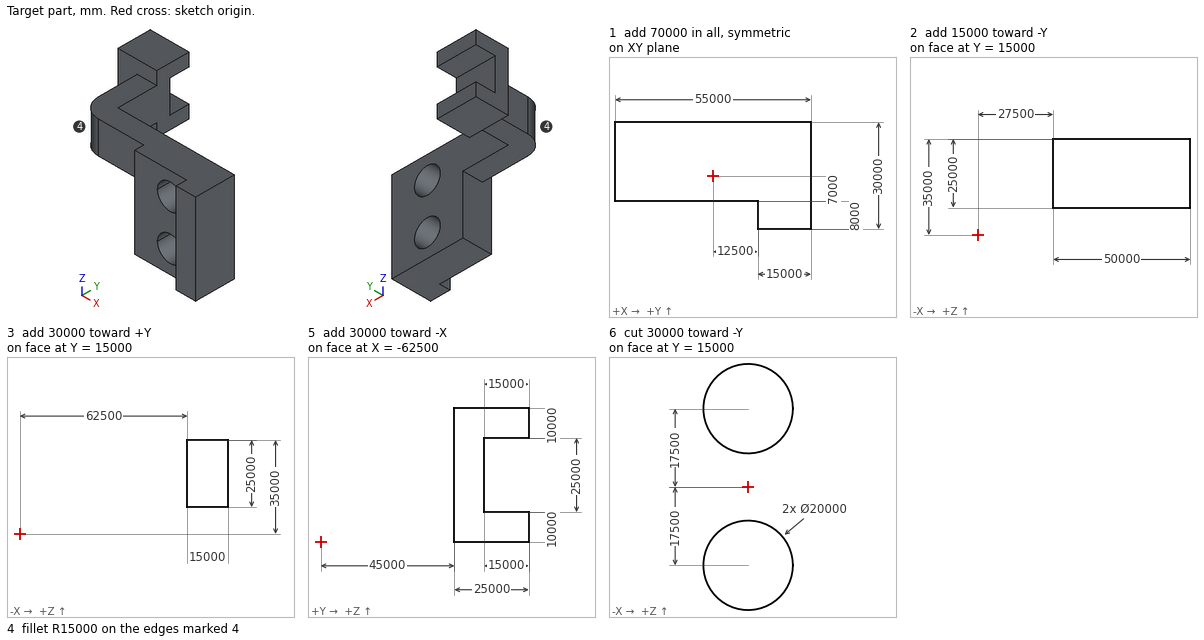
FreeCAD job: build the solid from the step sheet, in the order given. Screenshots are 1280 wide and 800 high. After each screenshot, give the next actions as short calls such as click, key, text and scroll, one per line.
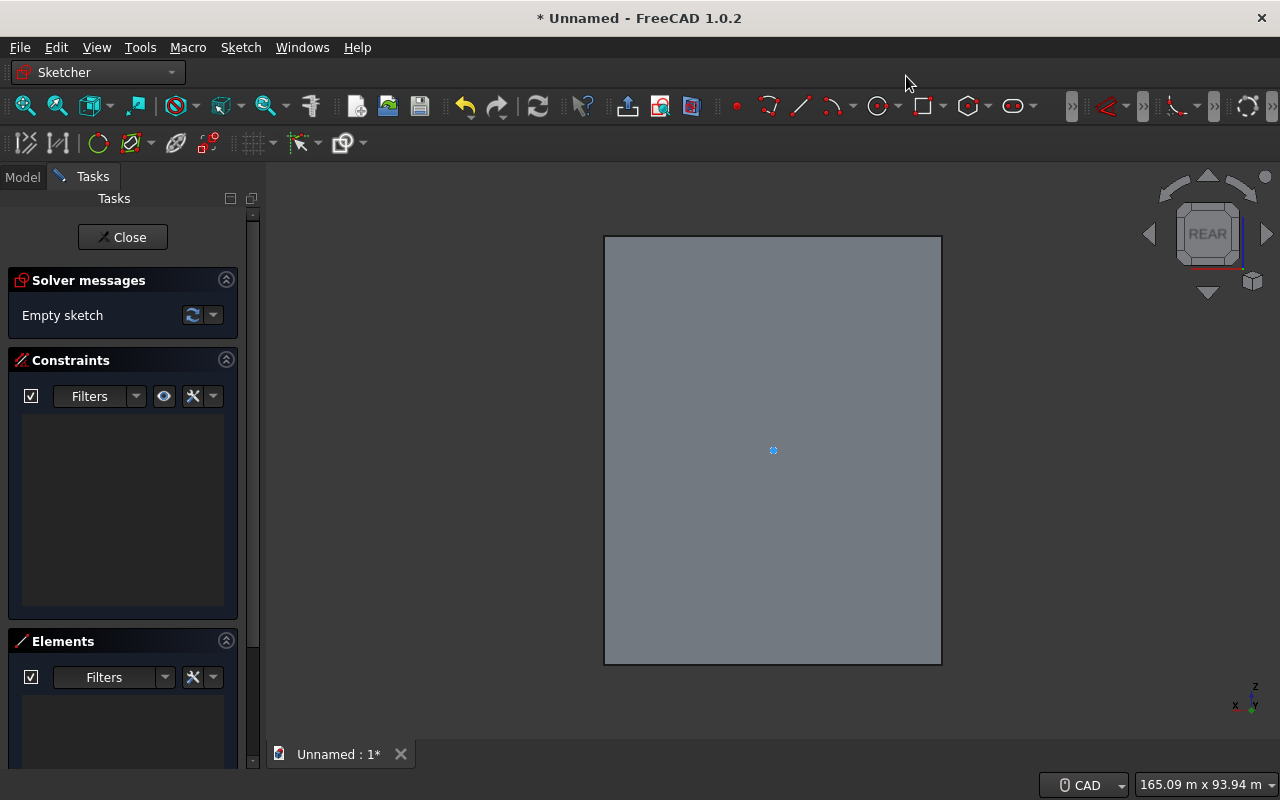
scroll(294, 711, down, 1)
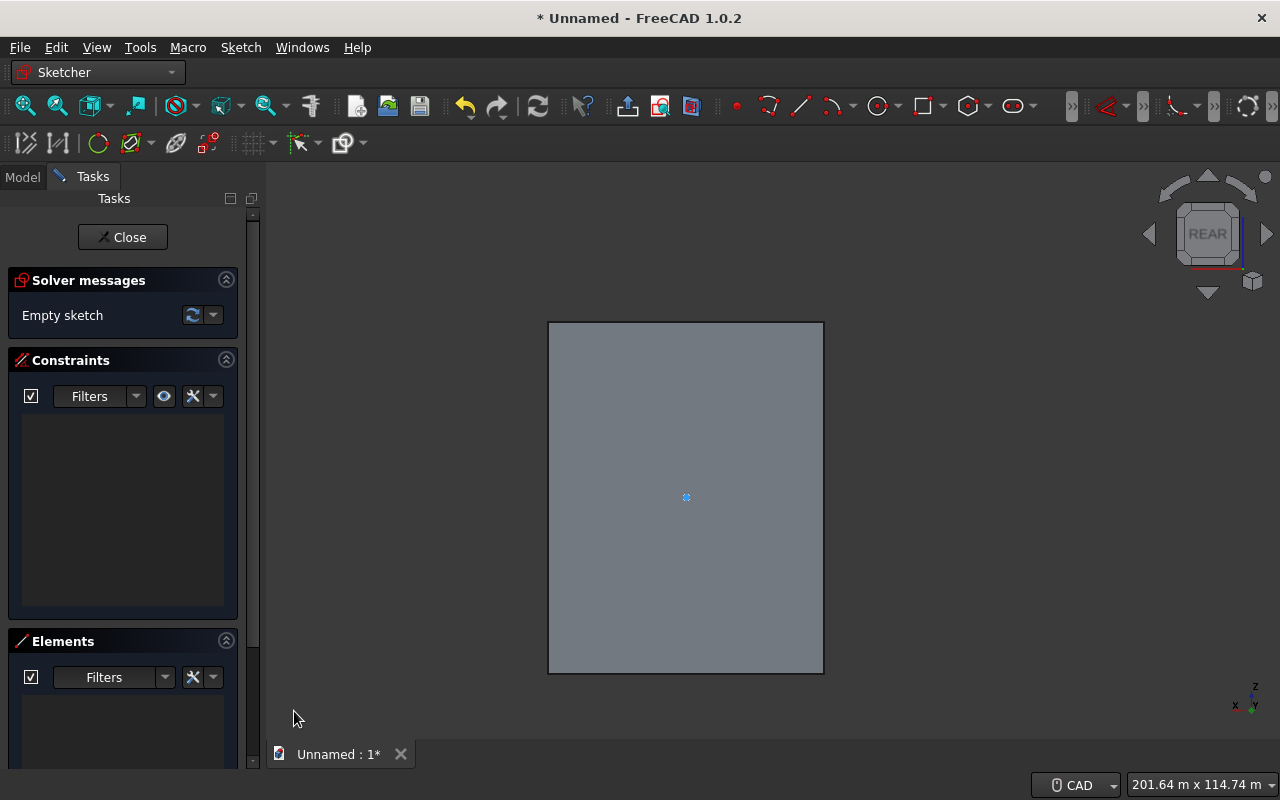
scroll(1115, 327, up, 2)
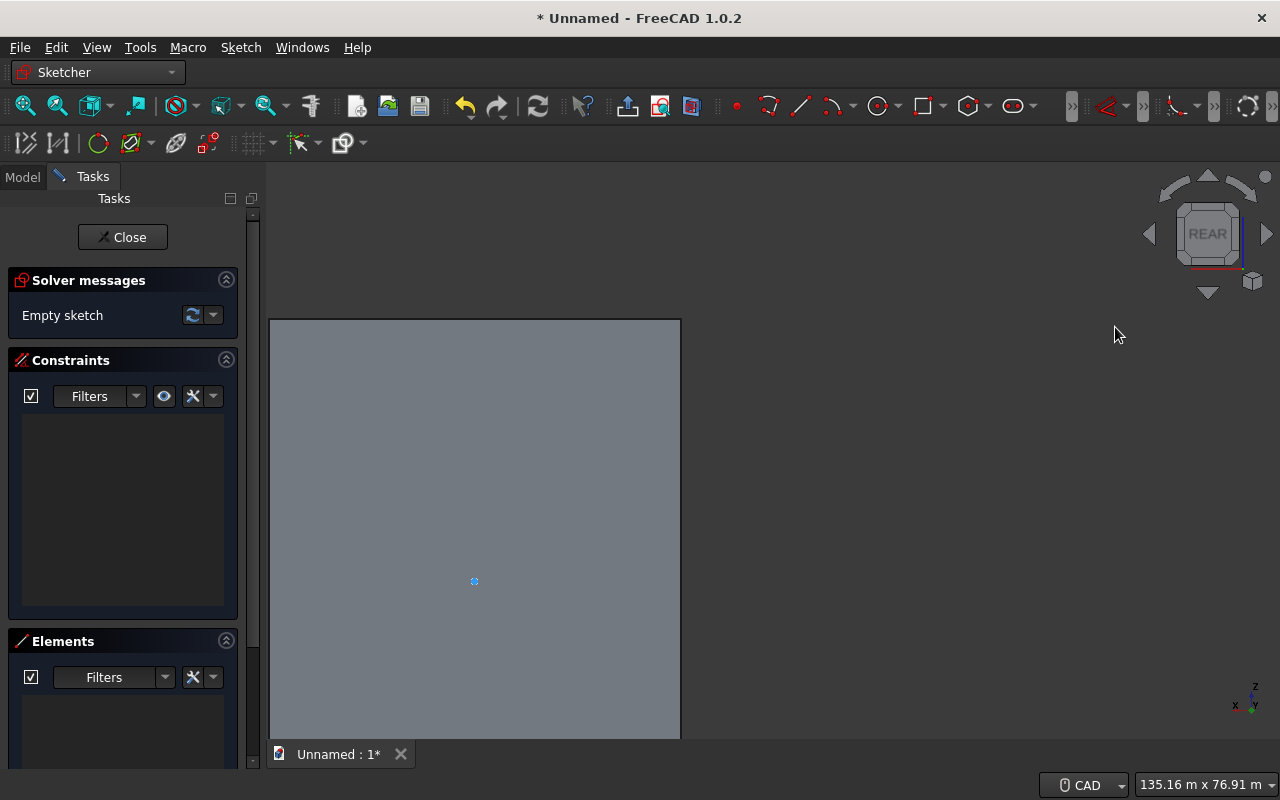
key(g)
key(r)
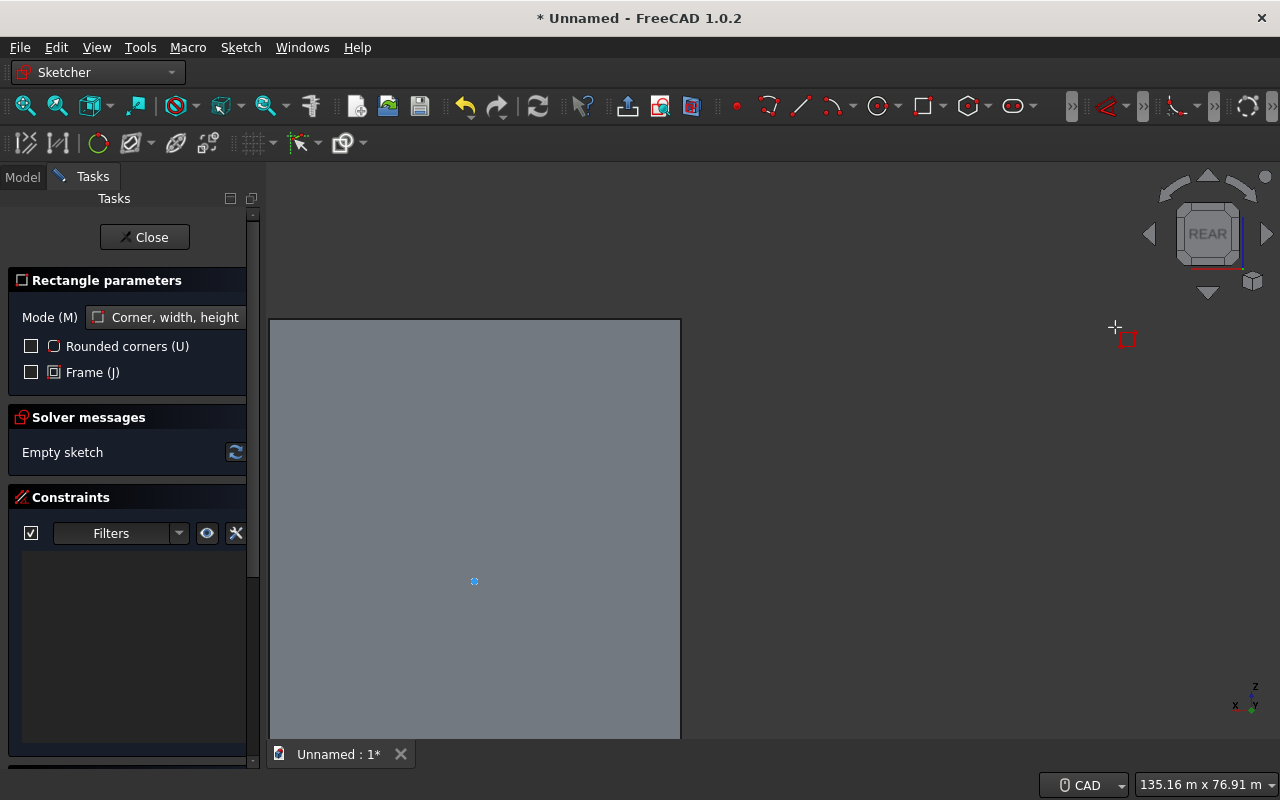
click(681, 319)
click(1056, 507)
key(Escape)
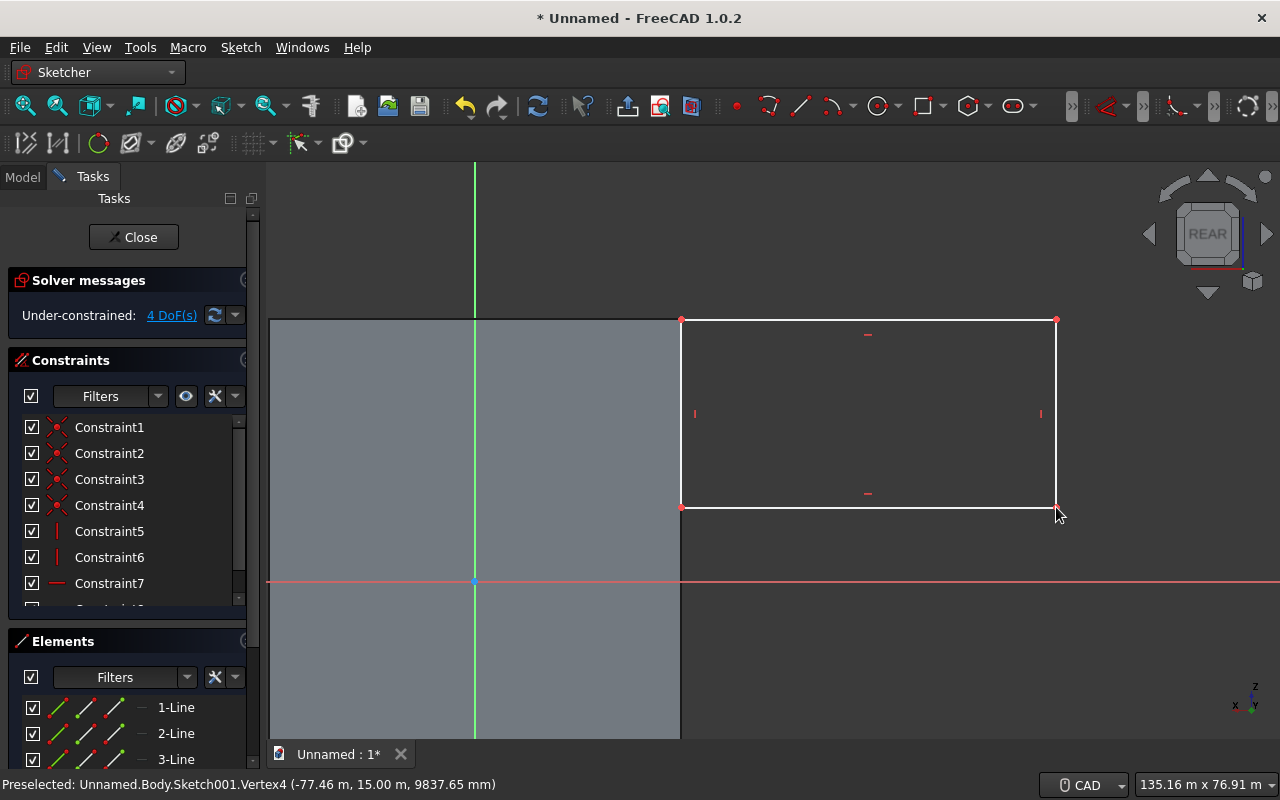
key(d)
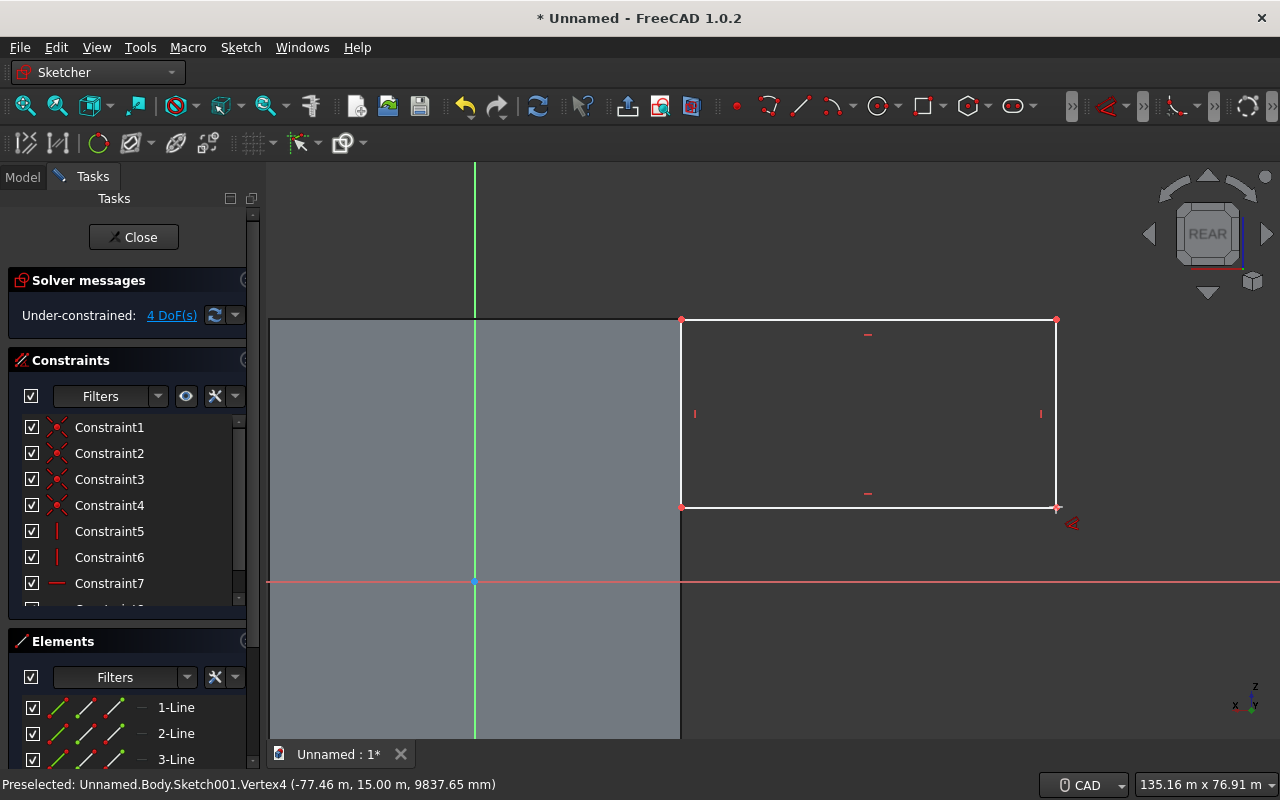
click(681, 376)
click(647, 414)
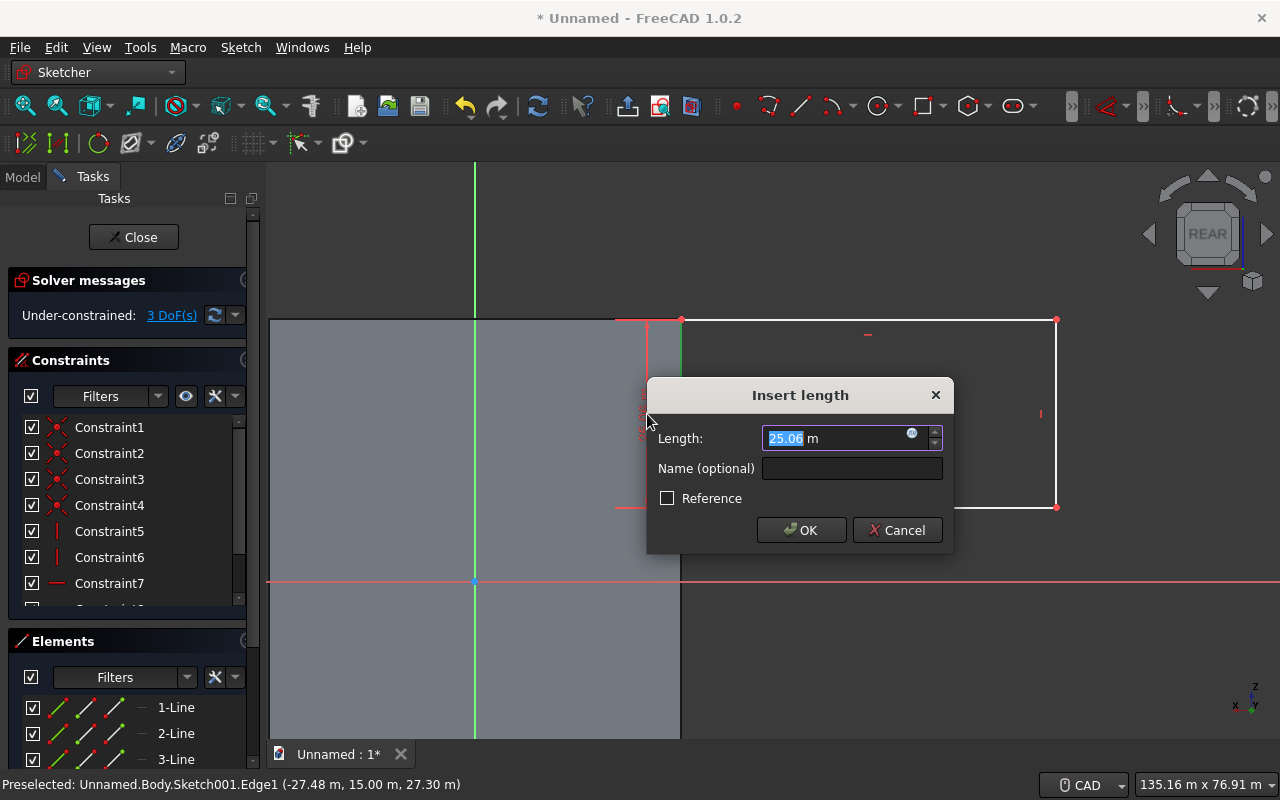
key(ctrl+a)
text(25000 mm)
key(Return)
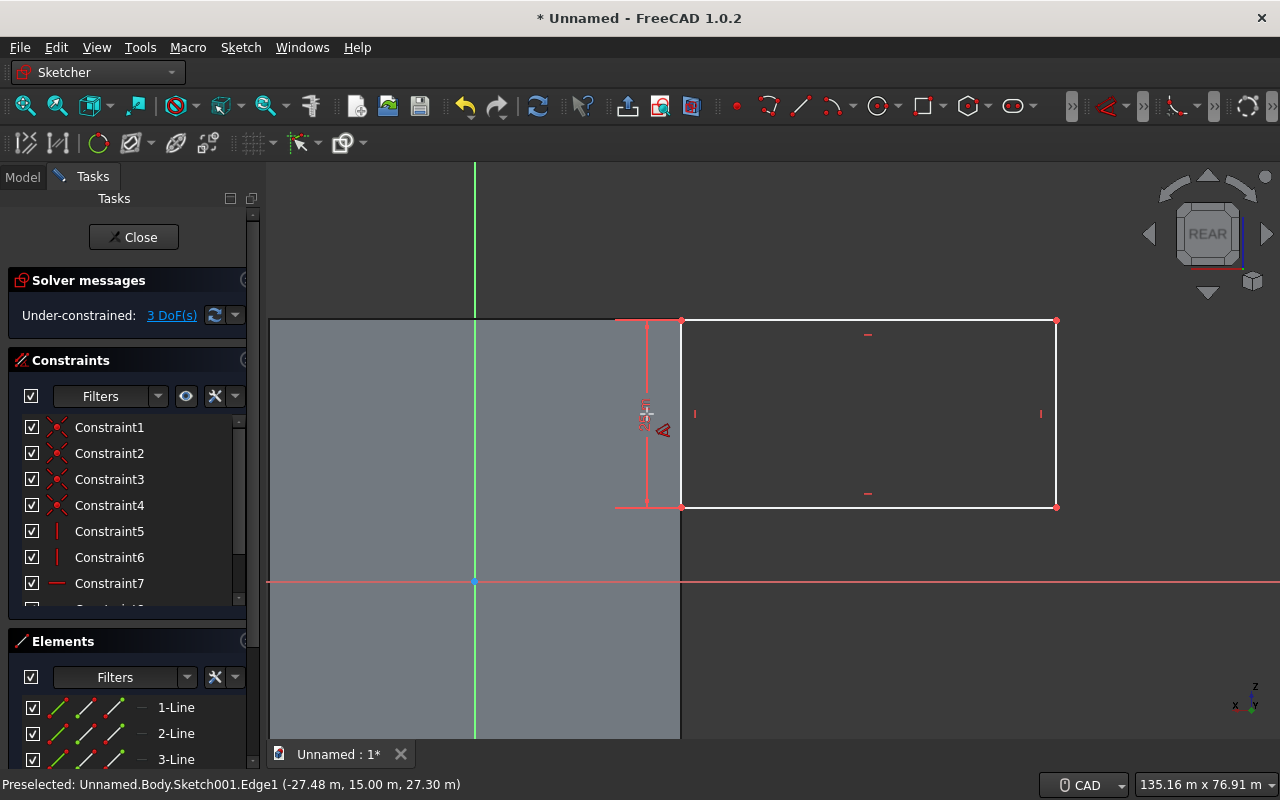
click(794, 508)
click(869, 542)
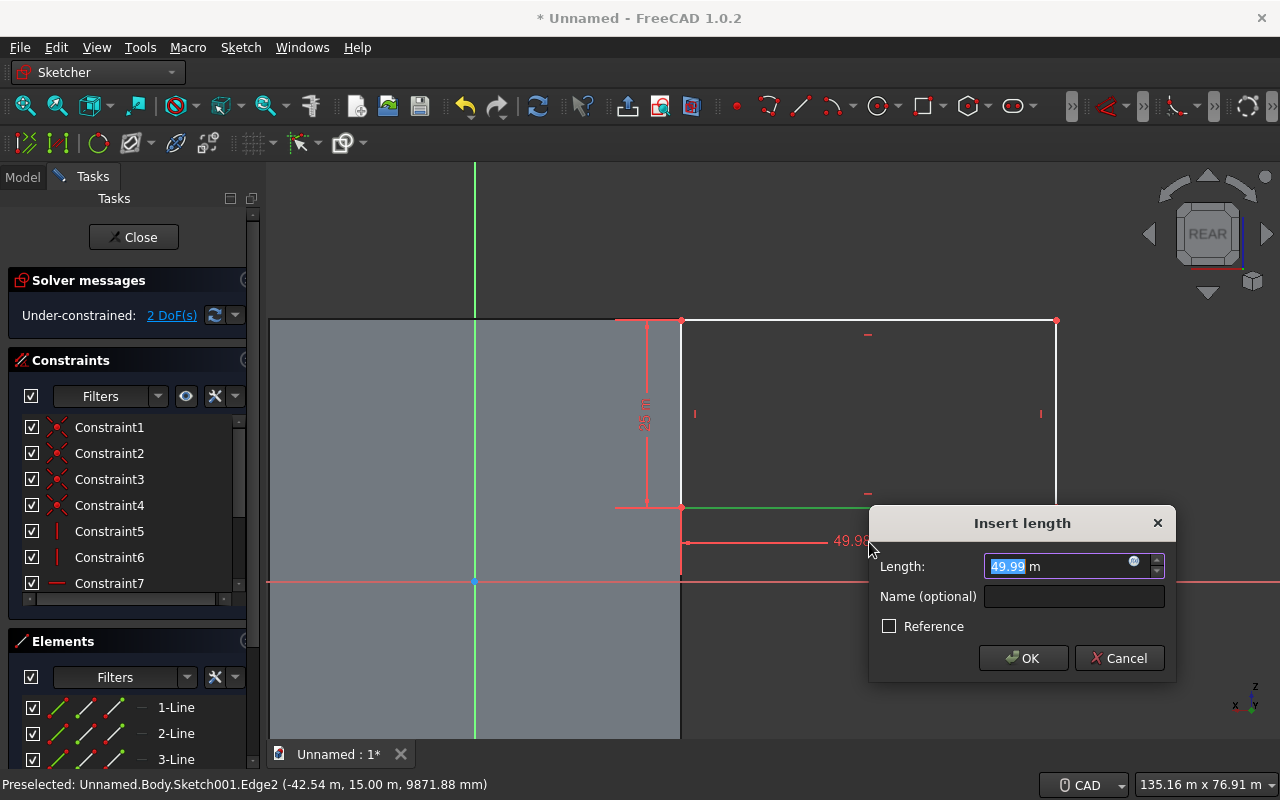
key(ctrl+a)
text(50000 mm)
key(Return)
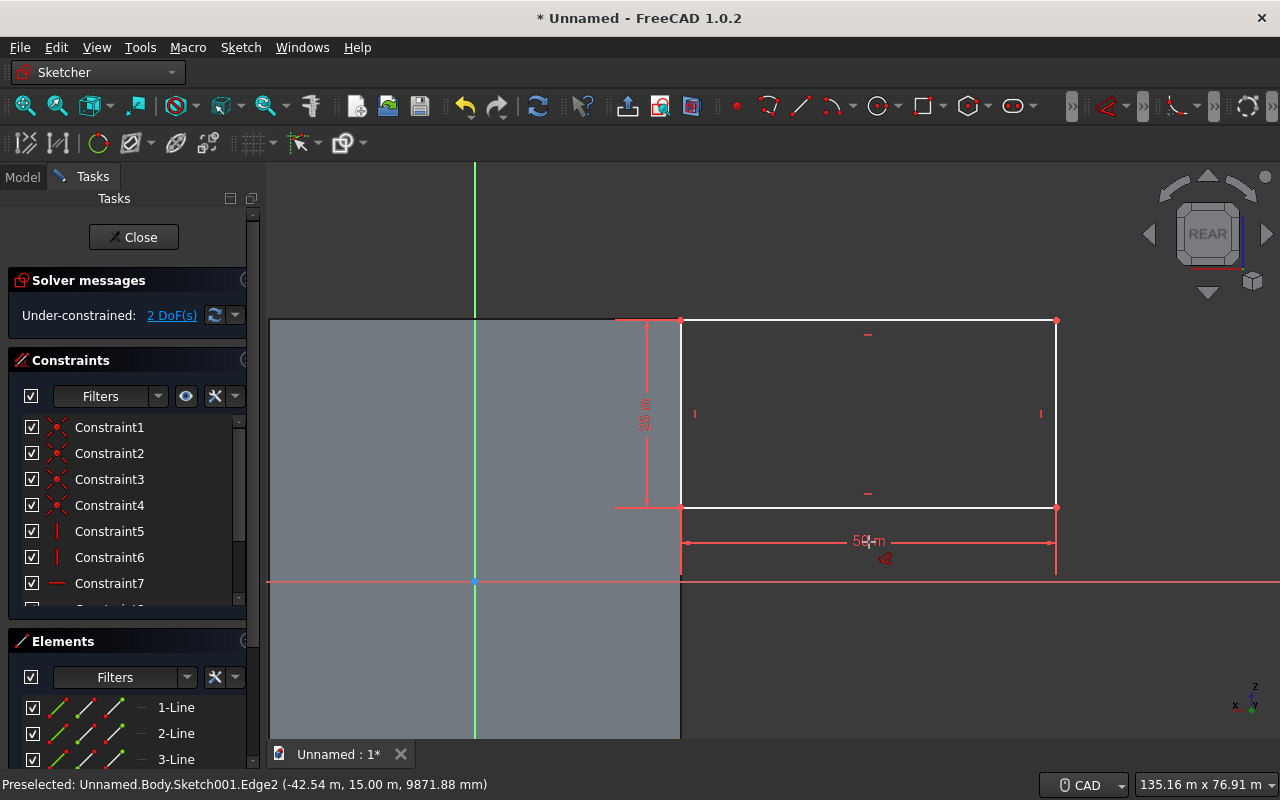
click(681, 320)
click(578, 616)